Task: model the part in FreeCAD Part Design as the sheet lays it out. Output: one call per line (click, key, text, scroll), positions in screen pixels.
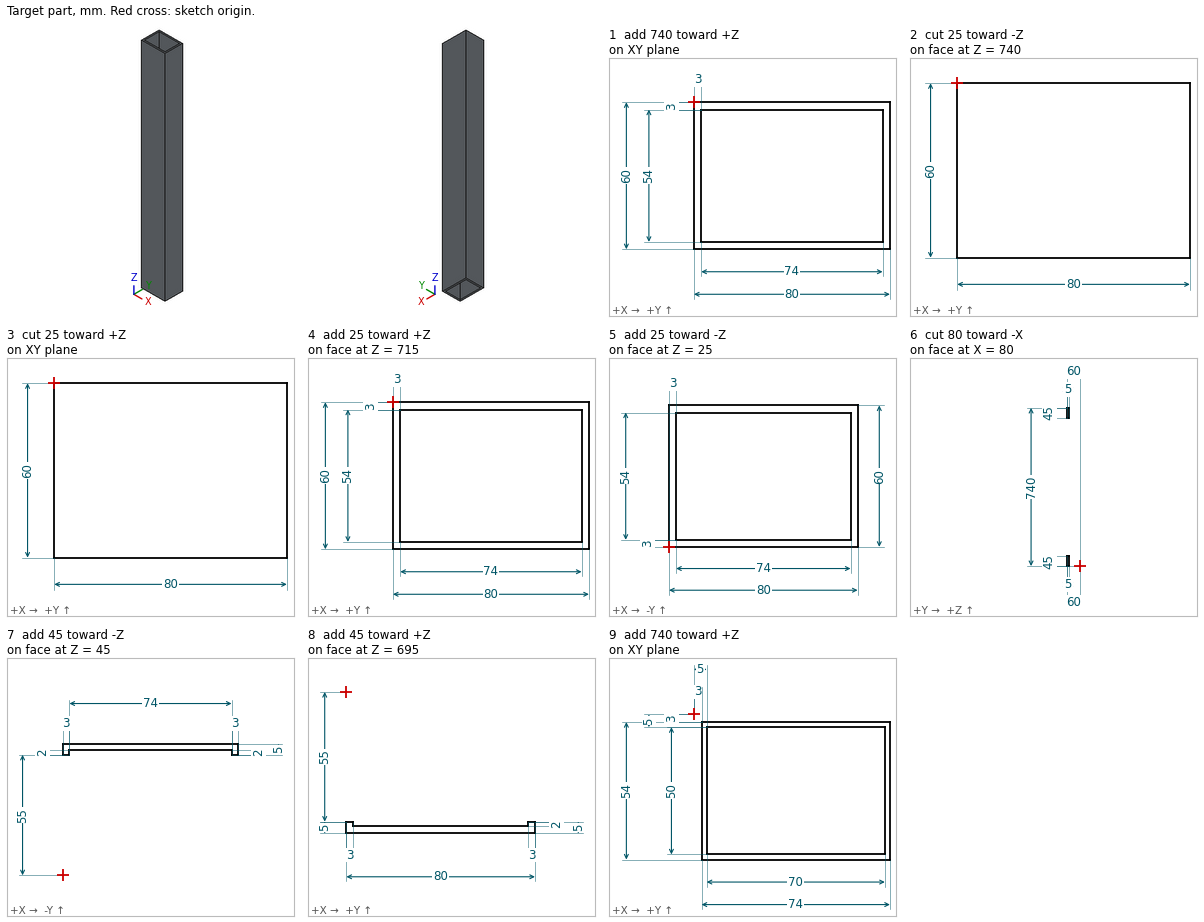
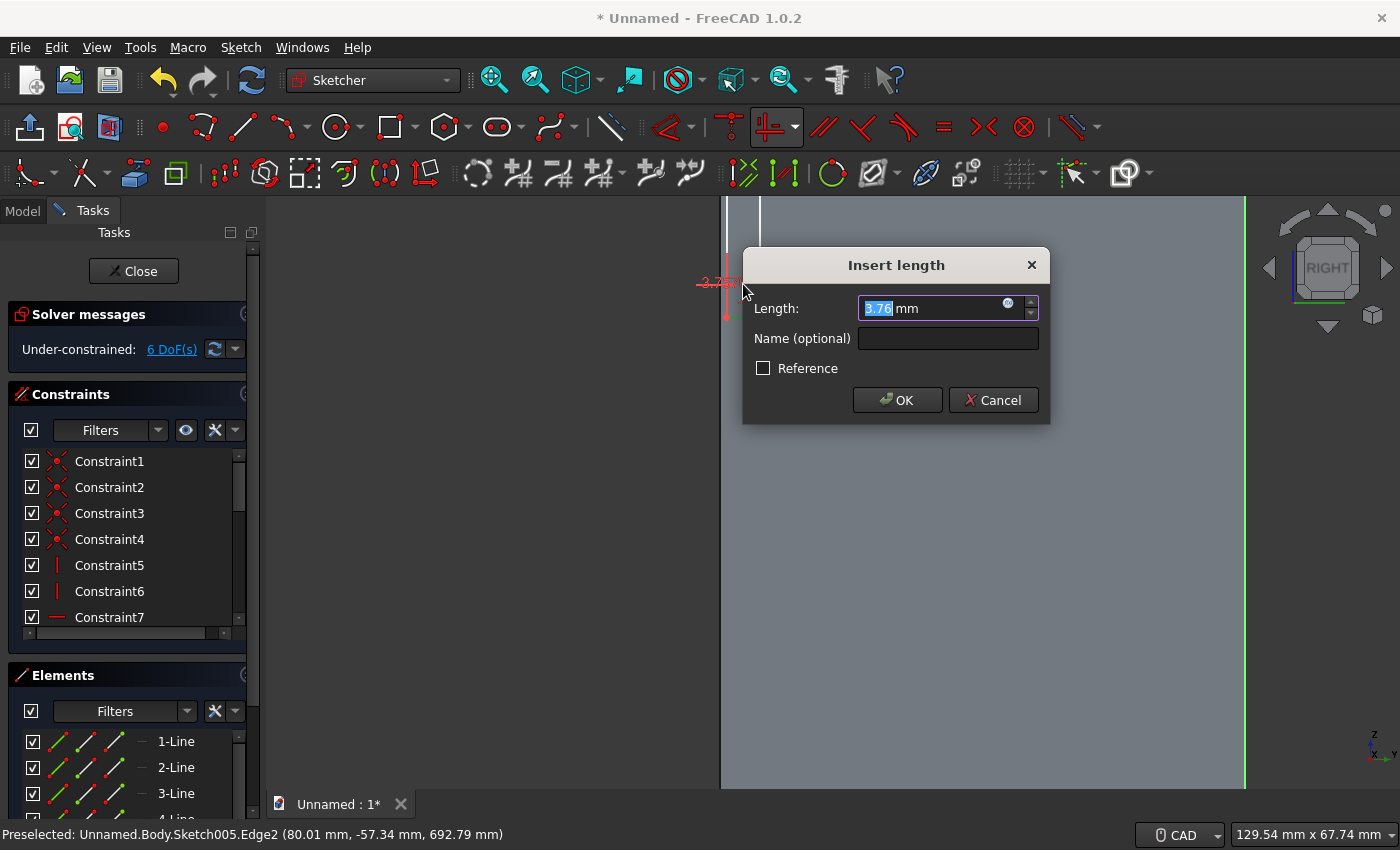
text(5)
key(Return)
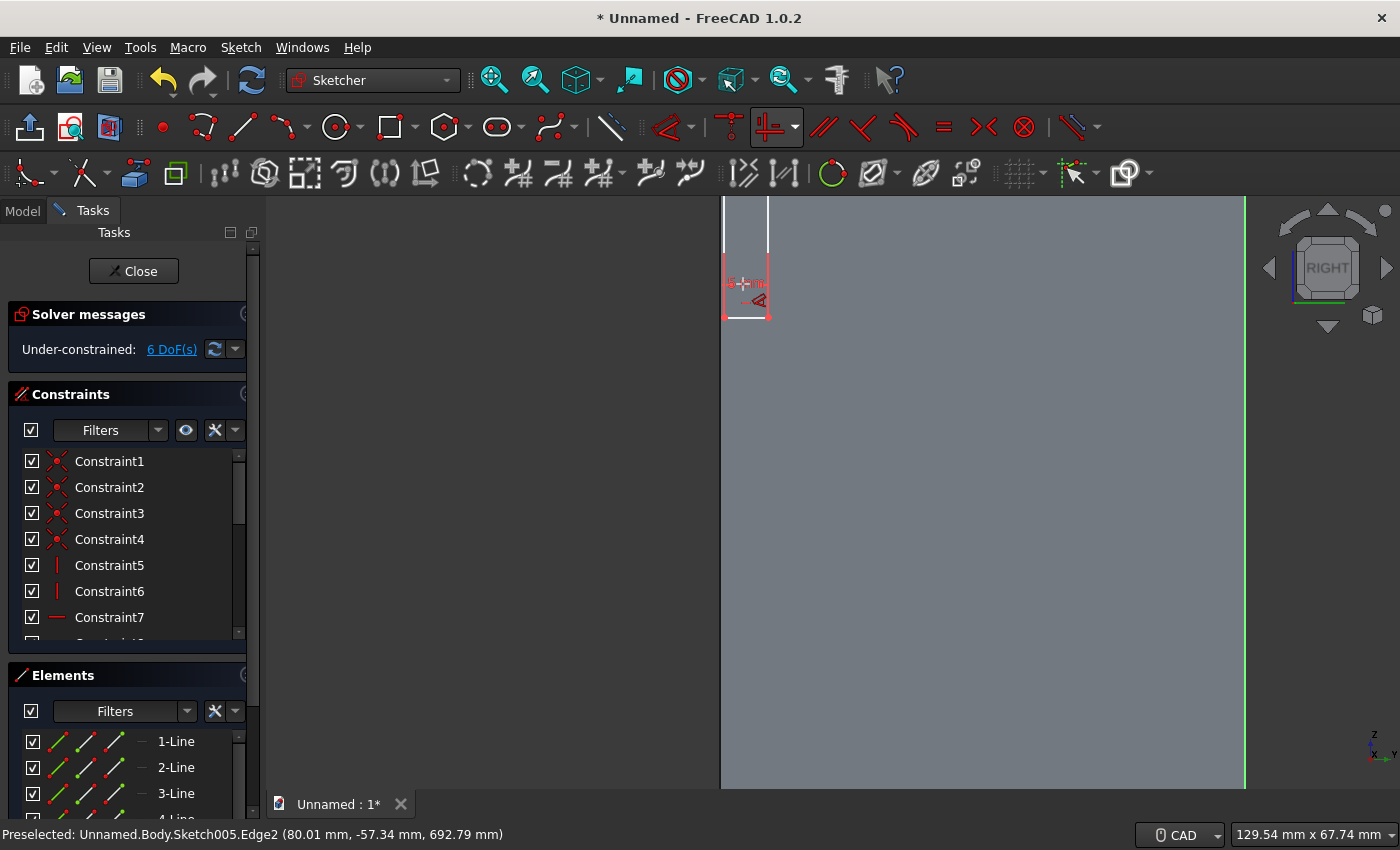
scroll(750, 321, down, 14)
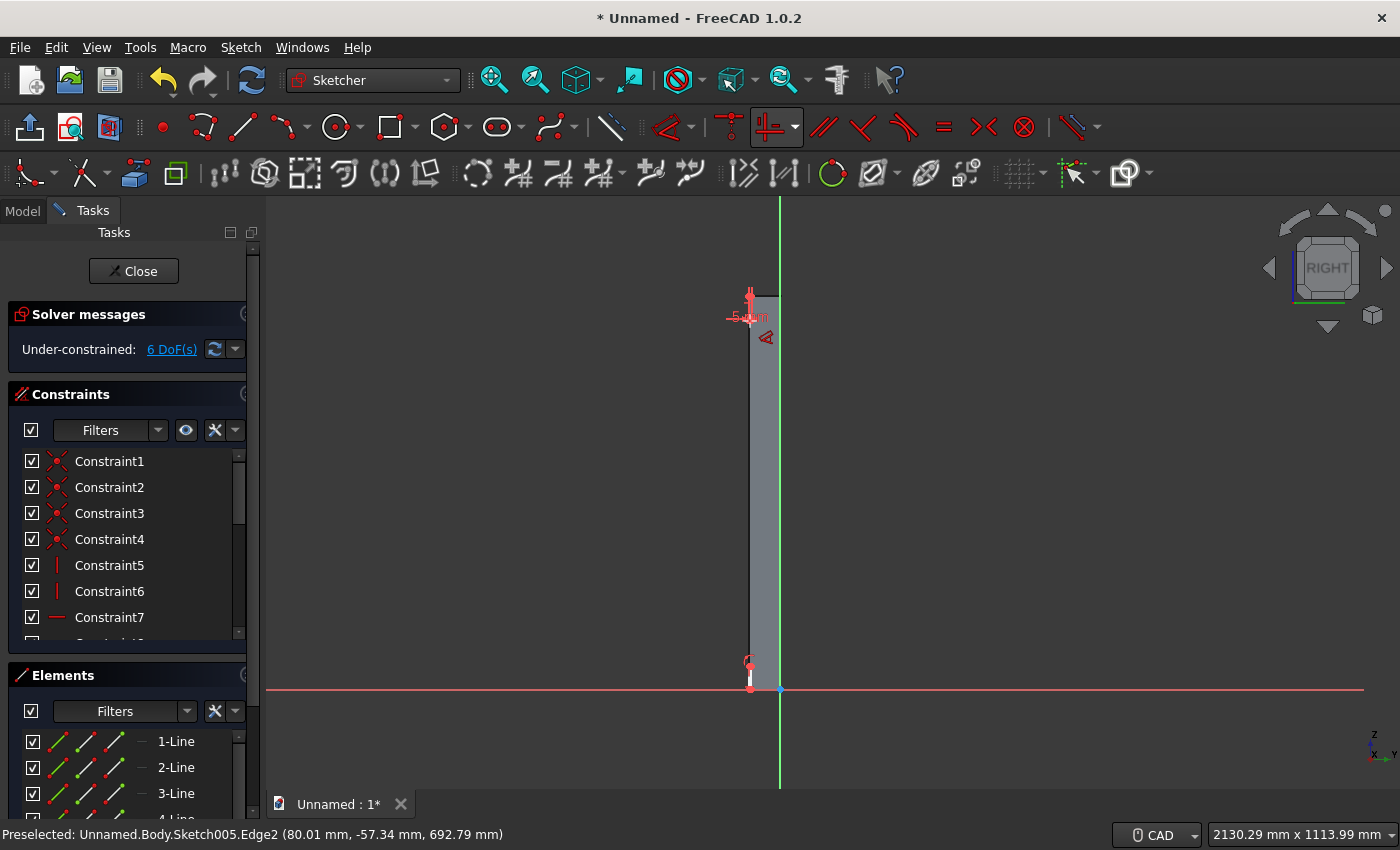
scroll(750, 690, up, 14)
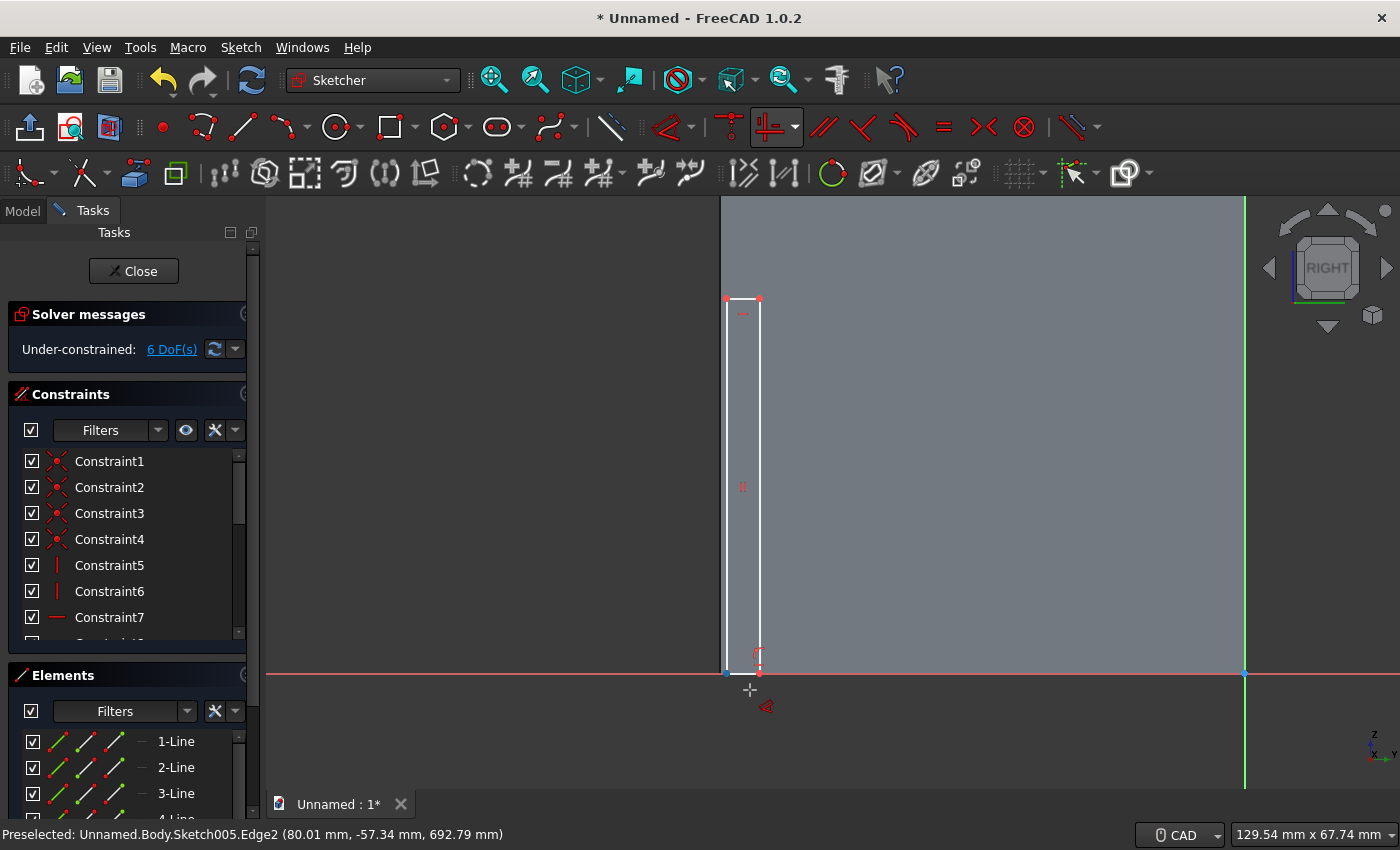
click(737, 674)
click(743, 708)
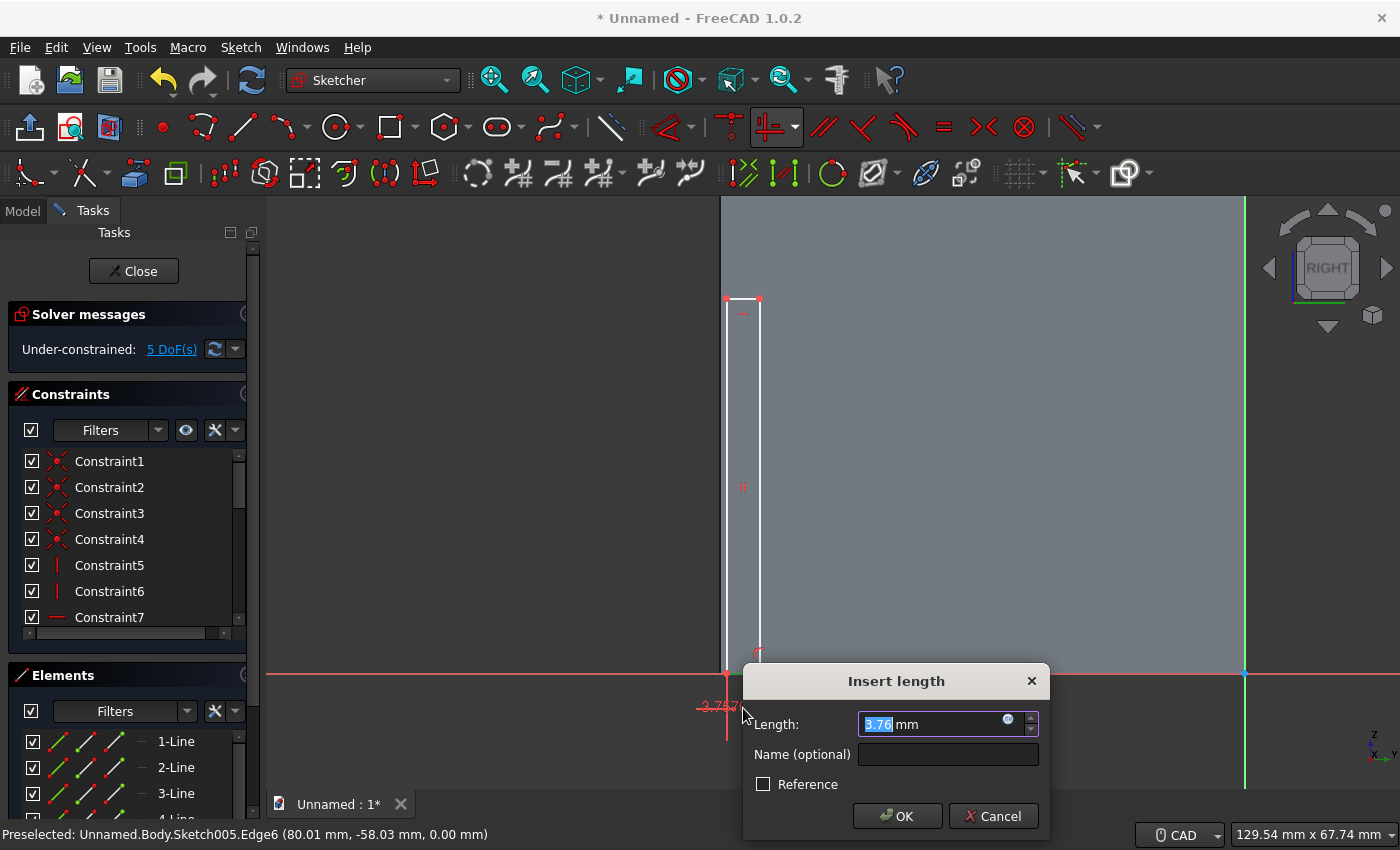
text(5)
key(Return)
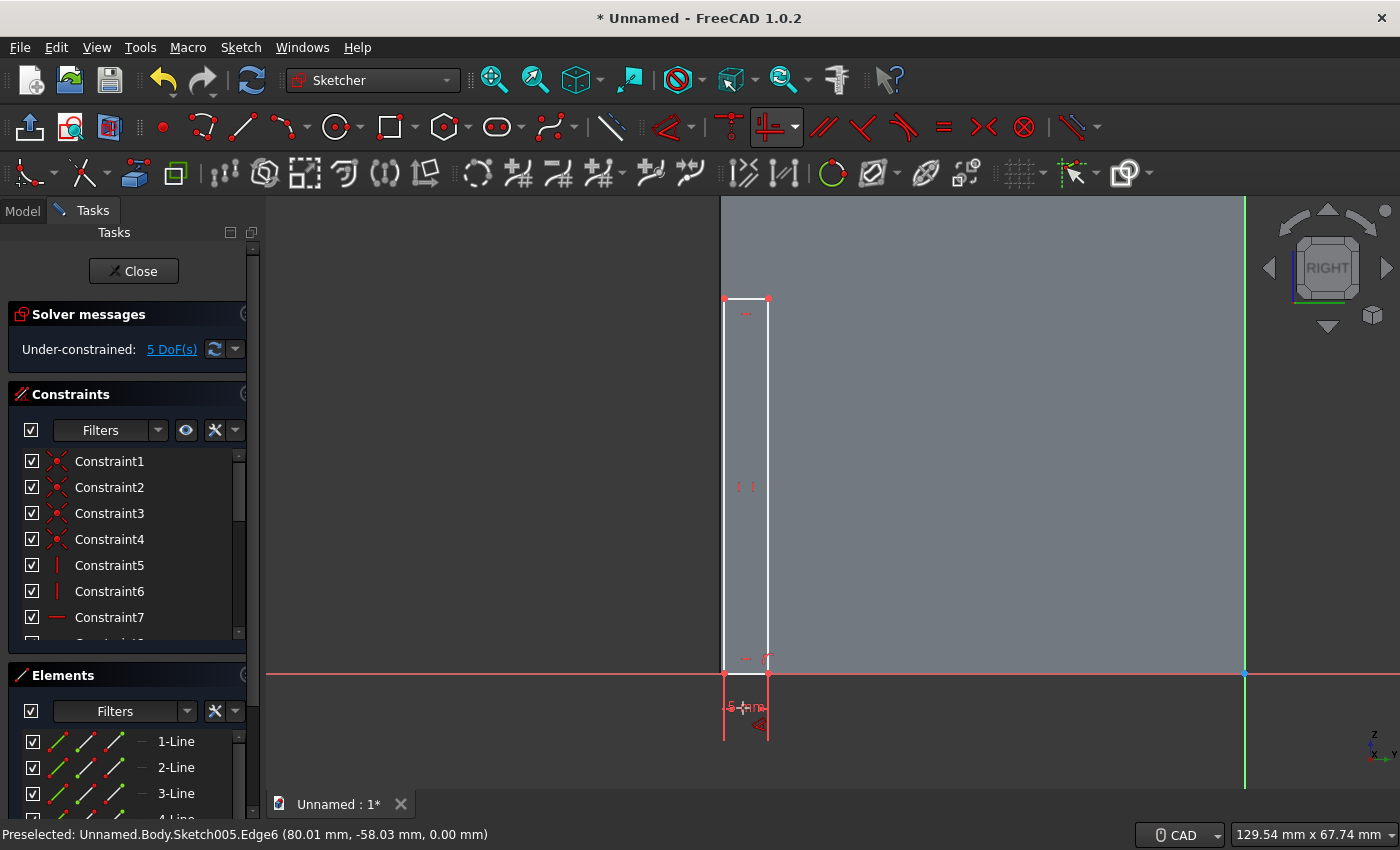
scroll(750, 690, down, 14)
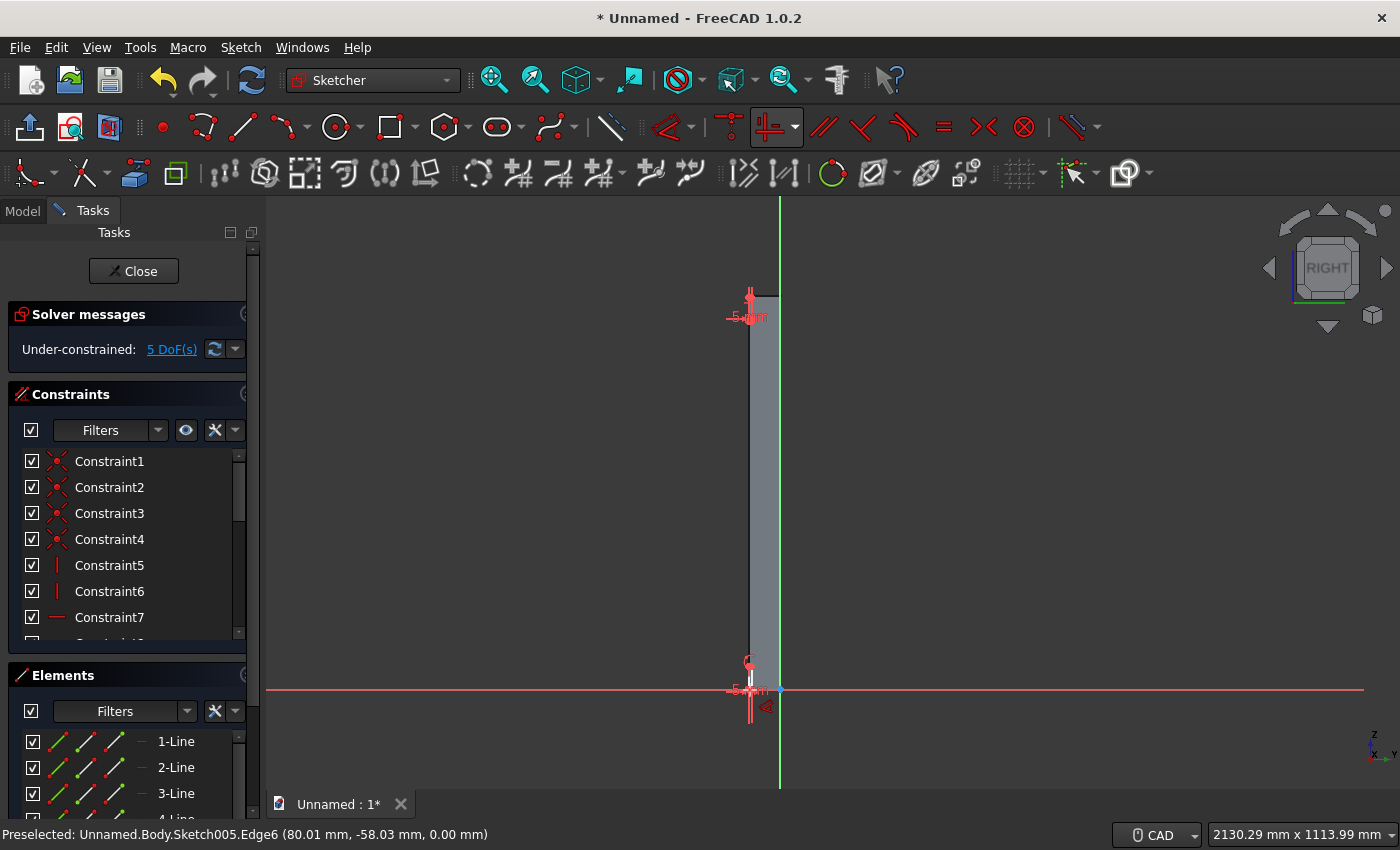
scroll(749, 304, up, 9)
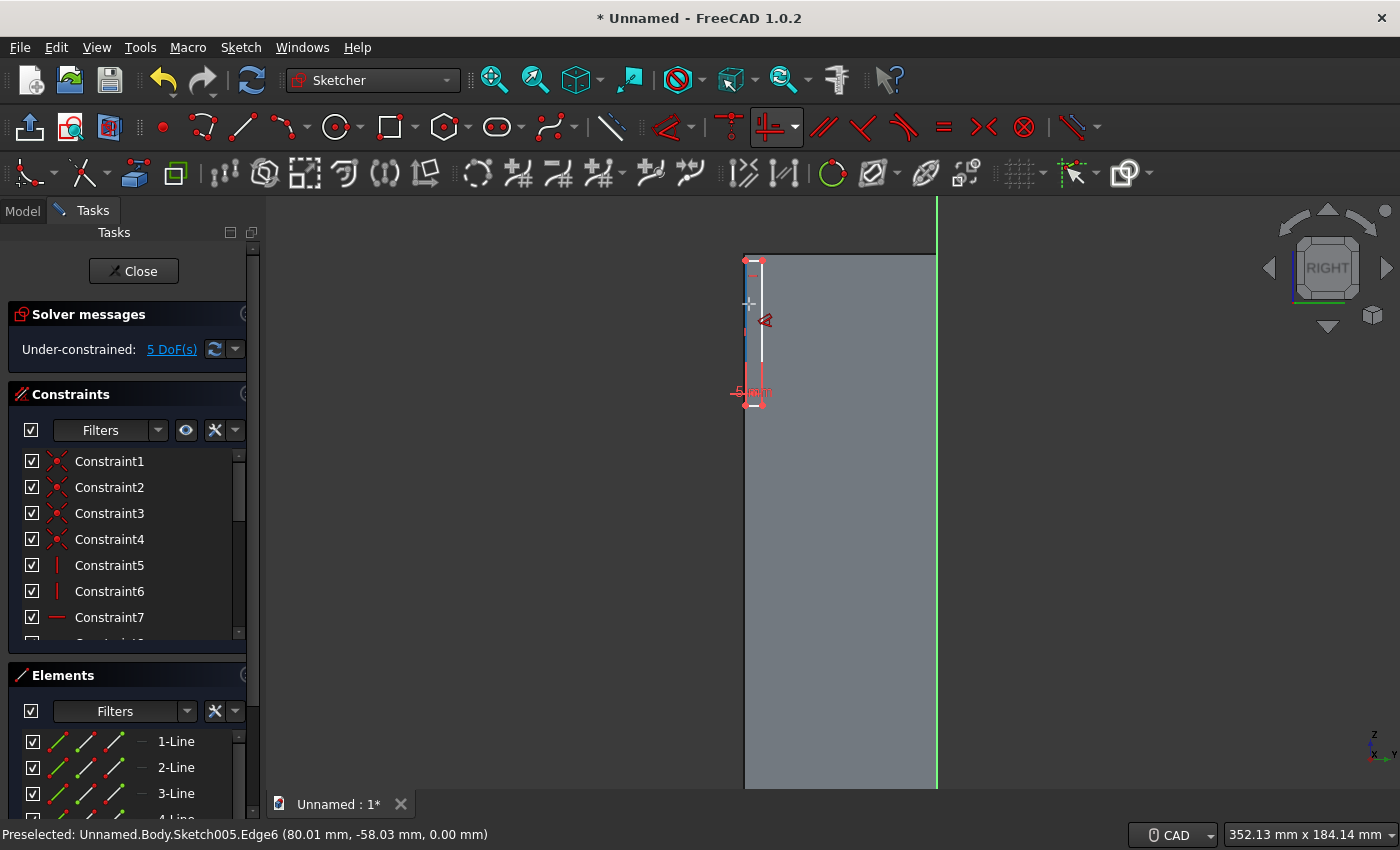
click(746, 304)
click(712, 333)